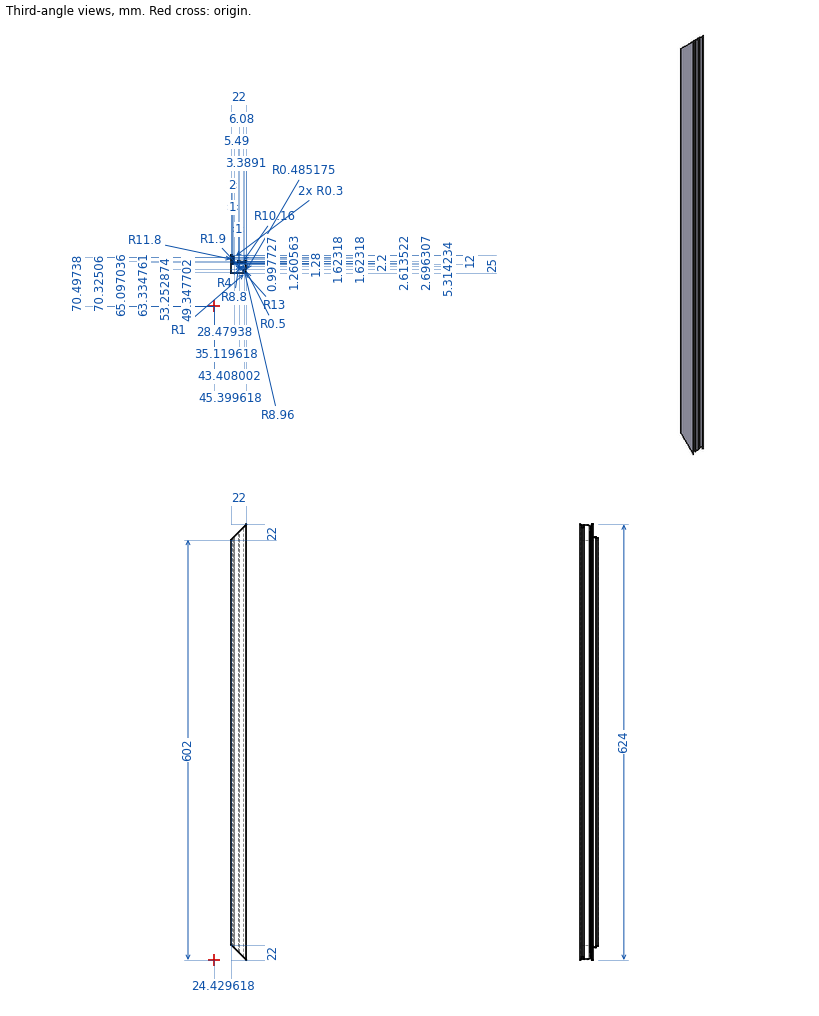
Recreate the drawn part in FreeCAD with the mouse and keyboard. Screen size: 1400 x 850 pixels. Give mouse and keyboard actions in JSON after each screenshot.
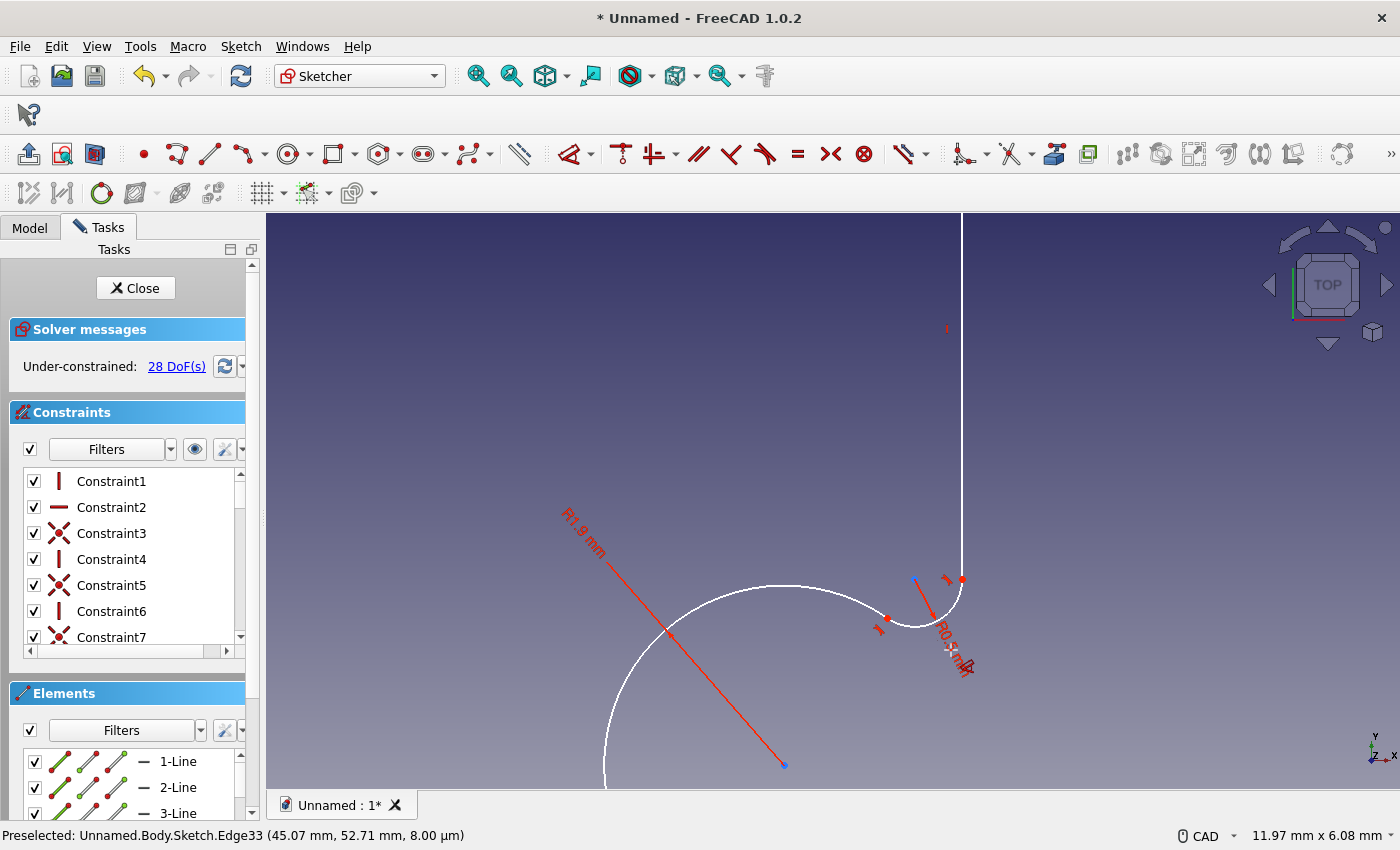
{"action": "scroll", "coordinate": [912, 627], "scroll_direction": "down", "scroll_amount": 9}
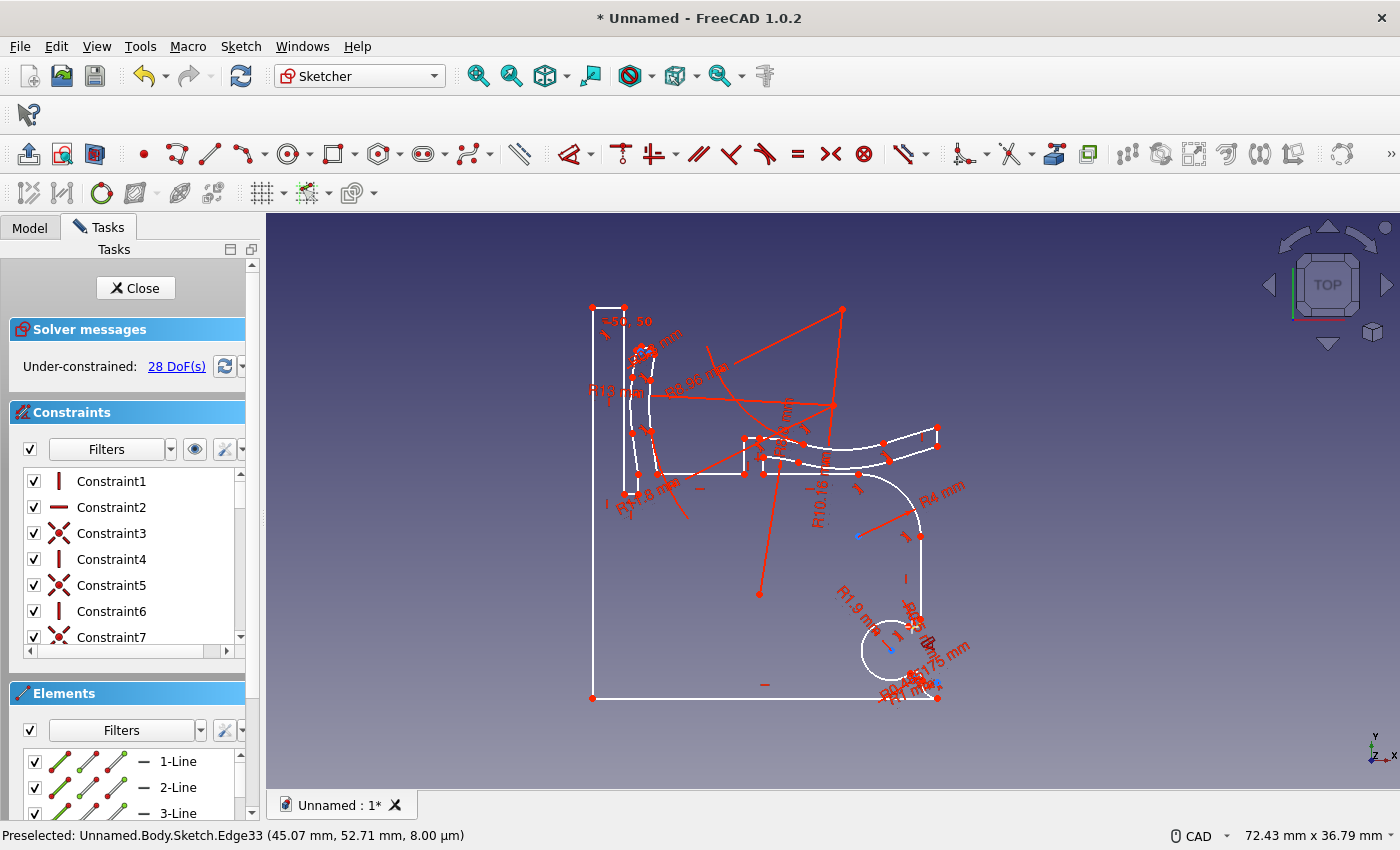
{"action": "scroll", "coordinate": [755, 438], "scroll_direction": "up", "scroll_amount": 6}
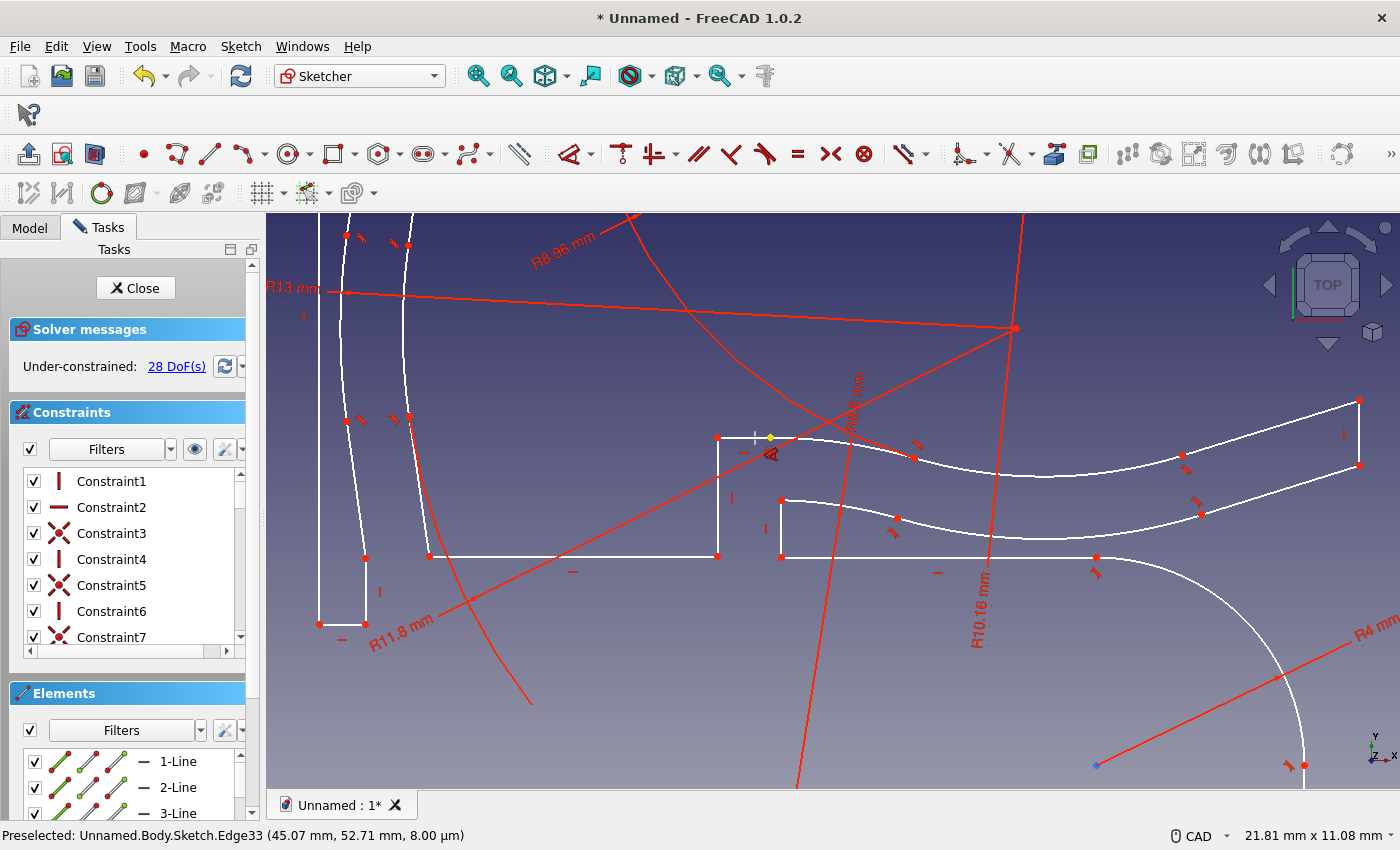
{"action": "left_click", "coordinate": [755, 438]}
{"action": "left_click", "coordinate": [744, 404]}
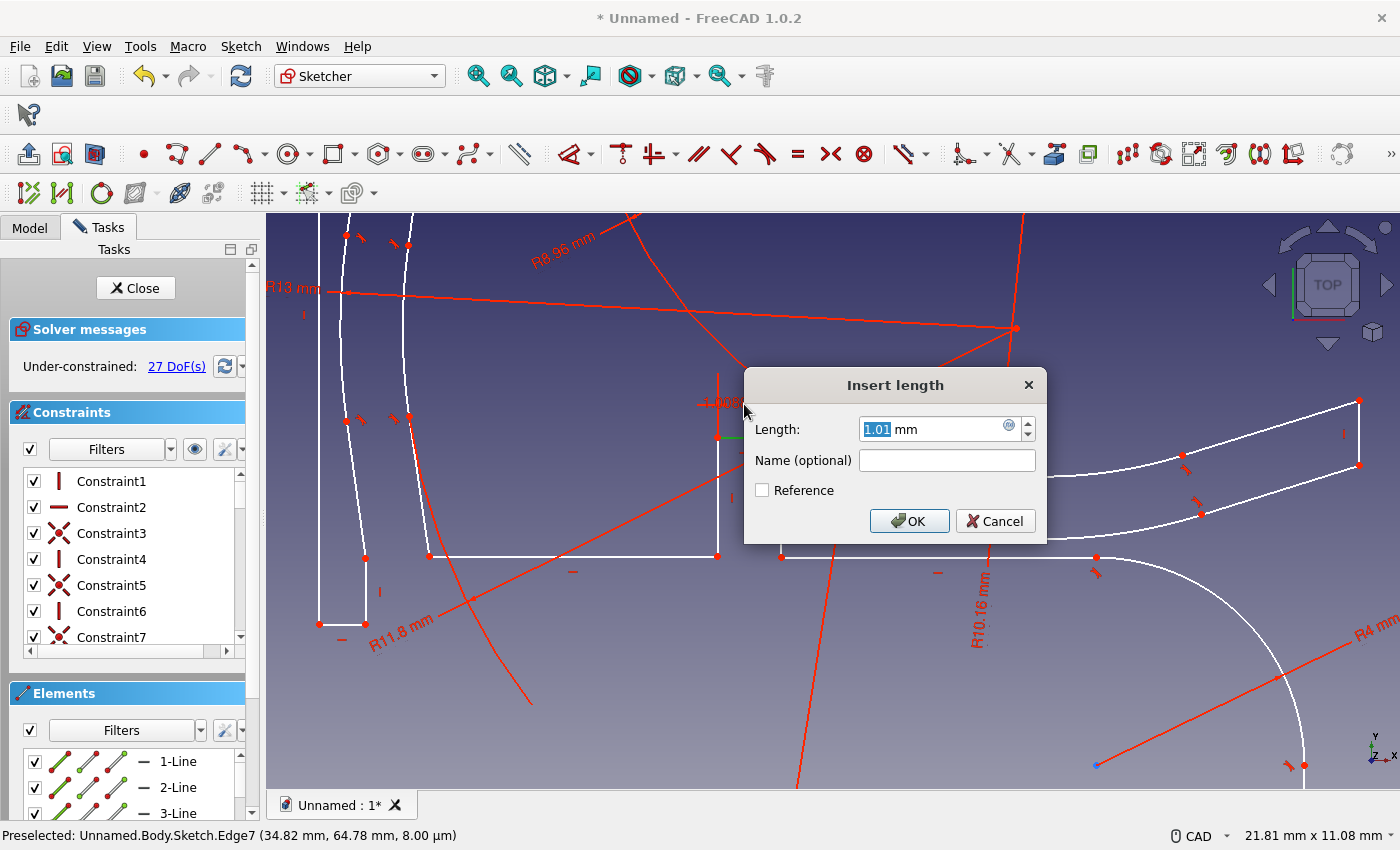
{"action": "type", "text": "1"}
{"action": "key", "text": "Return"}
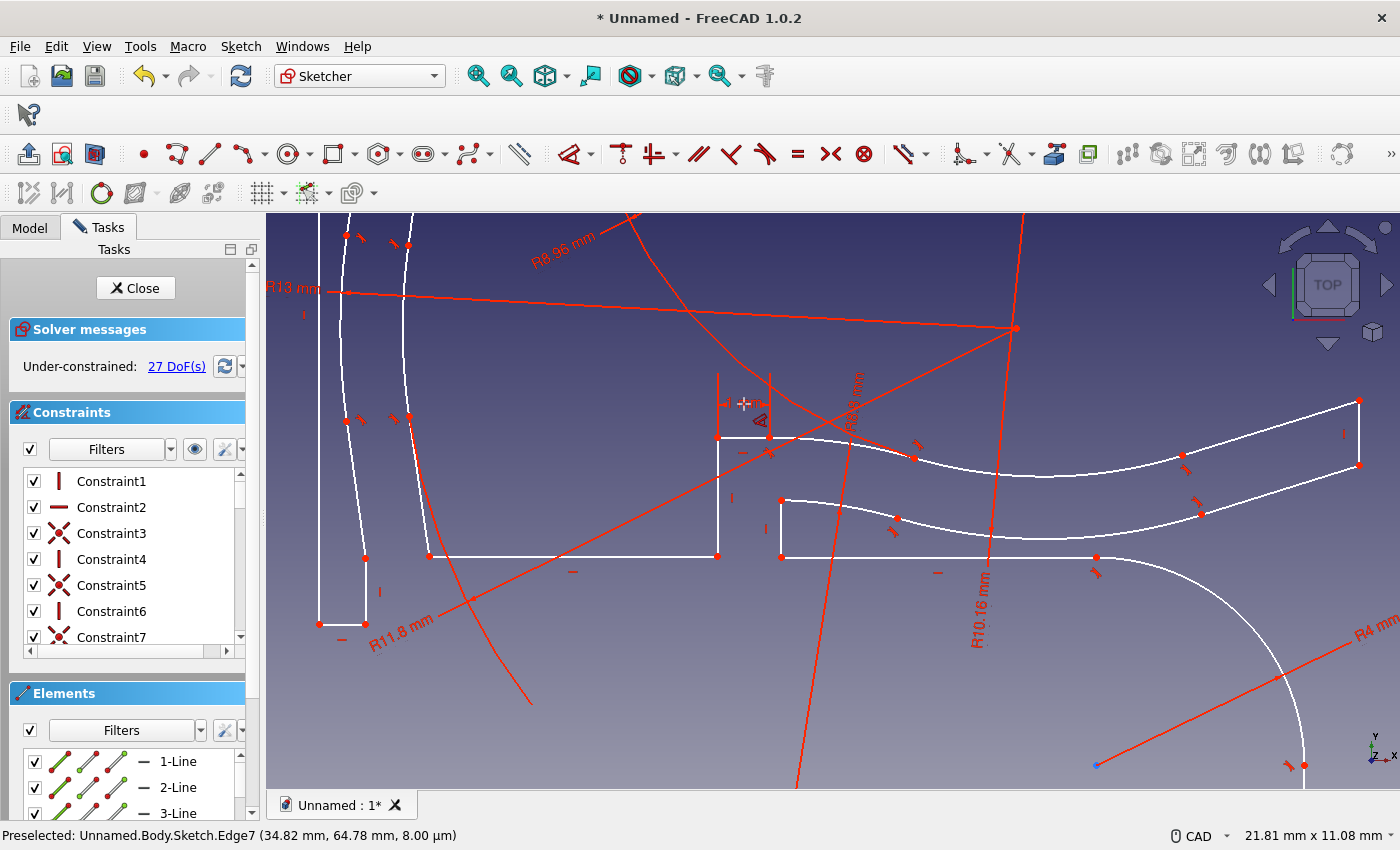
{"action": "left_click", "coordinate": [352, 625]}
{"action": "left_click", "coordinate": [342, 591]}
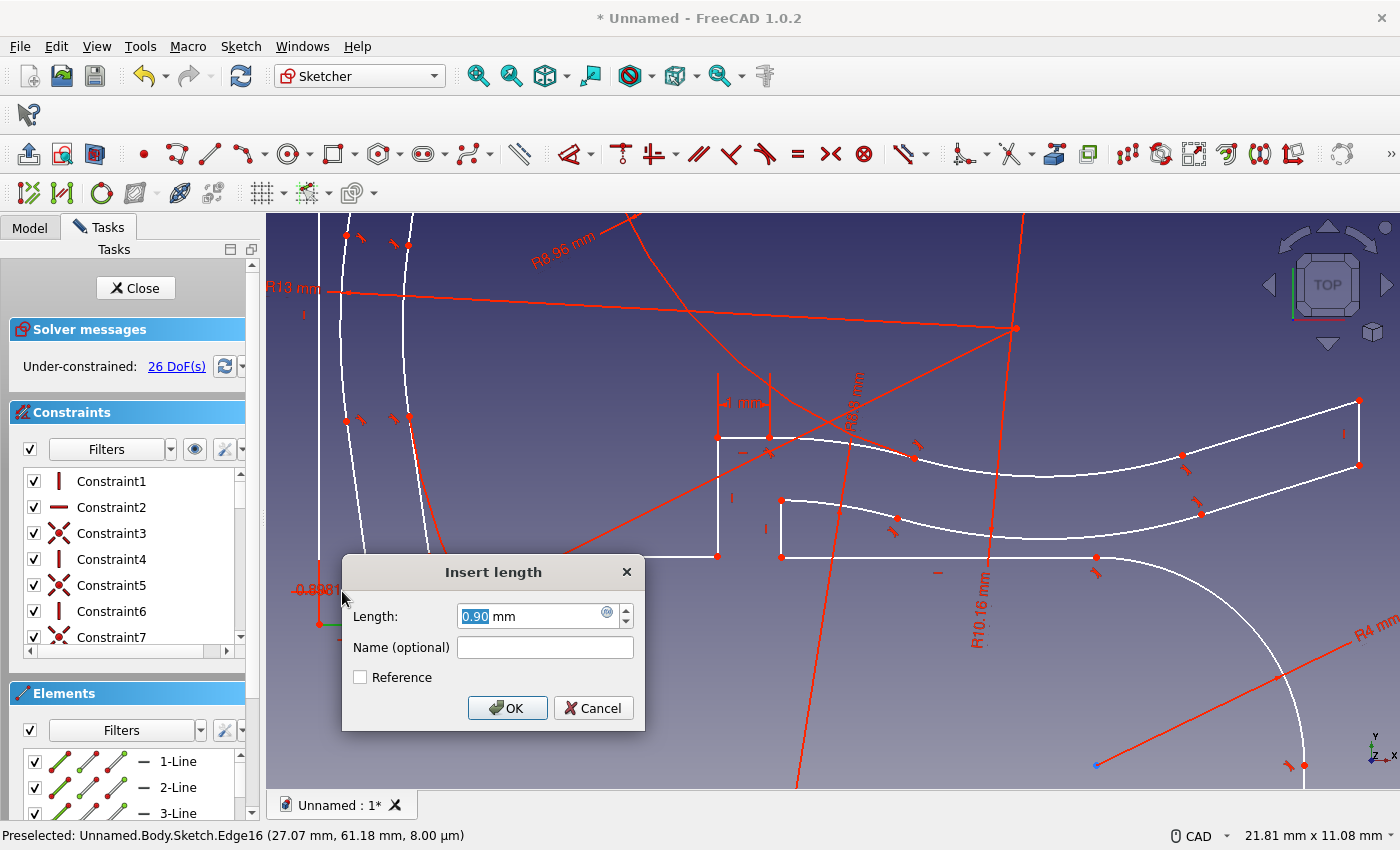
{"action": "type", "text": "1"}
{"action": "key", "text": "Return"}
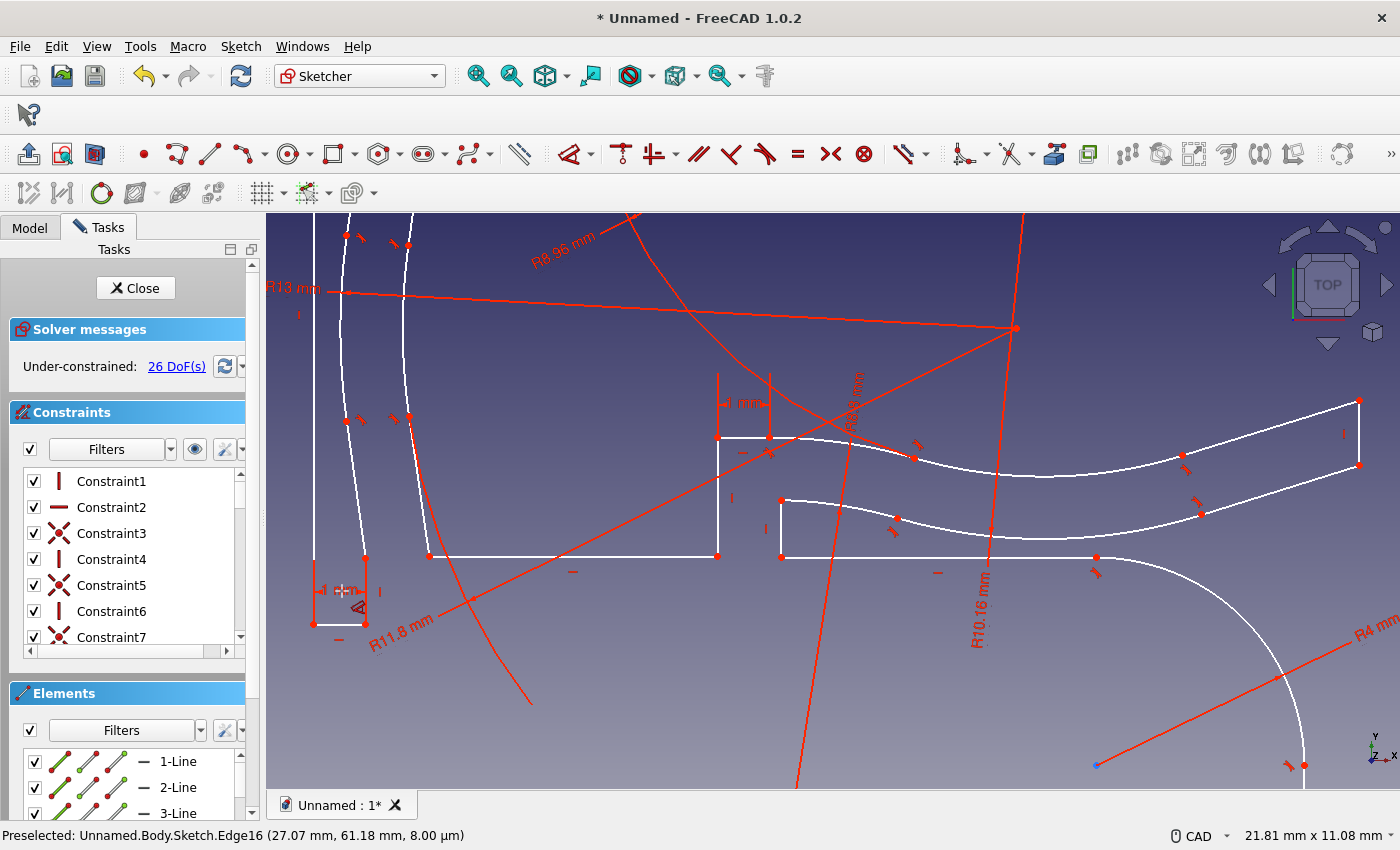
{"action": "scroll", "coordinate": [755, 437], "scroll_direction": "down", "scroll_amount": 6}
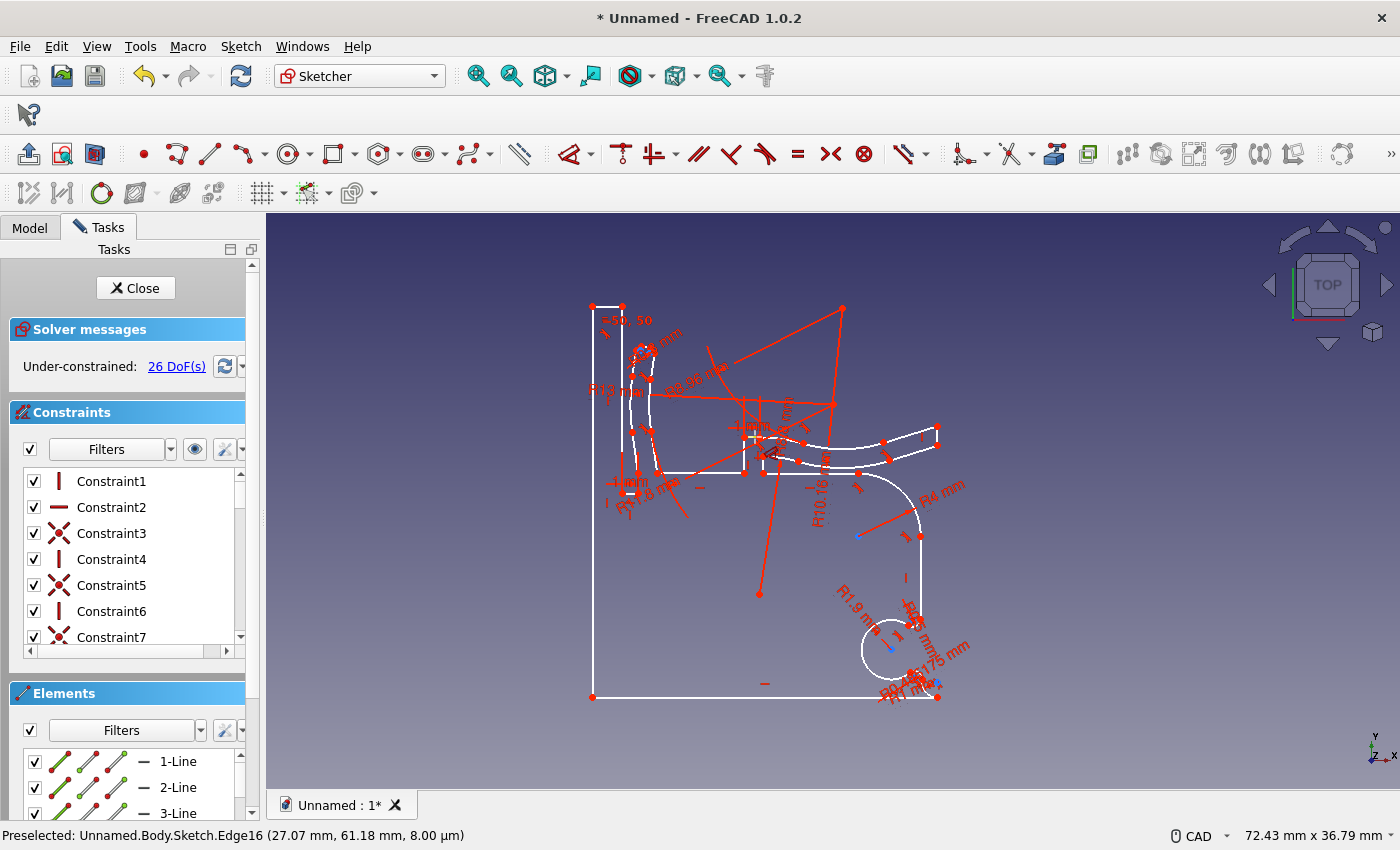
{"action": "scroll", "coordinate": [614, 307], "scroll_direction": "up", "scroll_amount": 3}